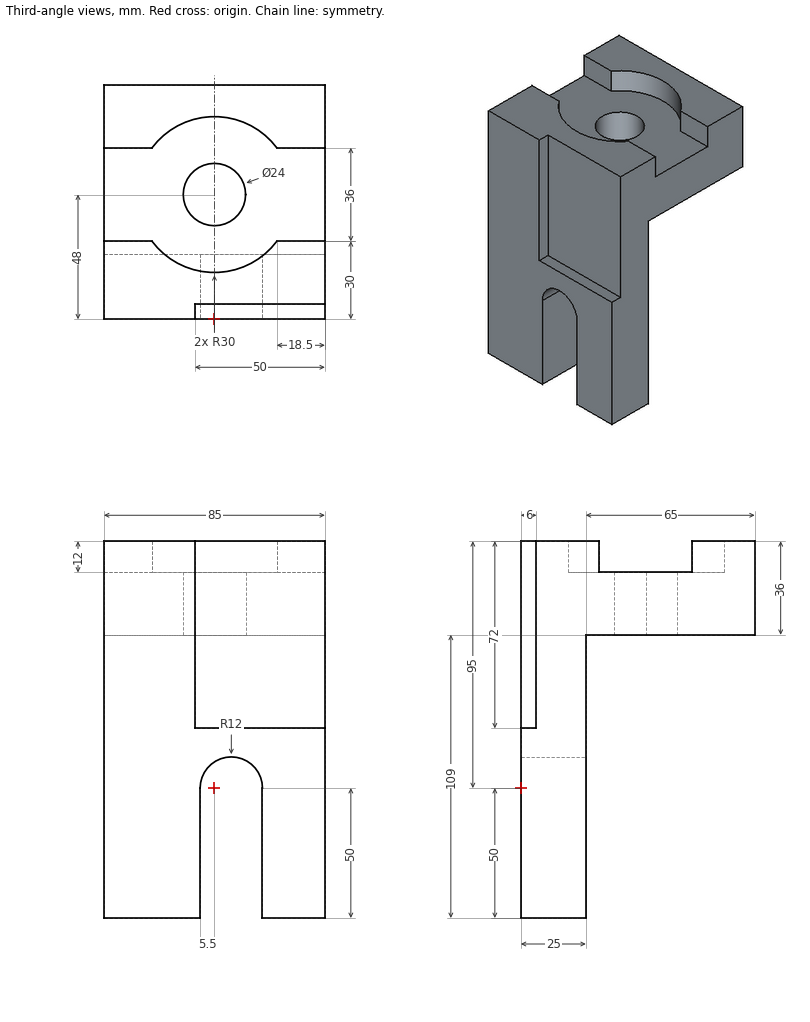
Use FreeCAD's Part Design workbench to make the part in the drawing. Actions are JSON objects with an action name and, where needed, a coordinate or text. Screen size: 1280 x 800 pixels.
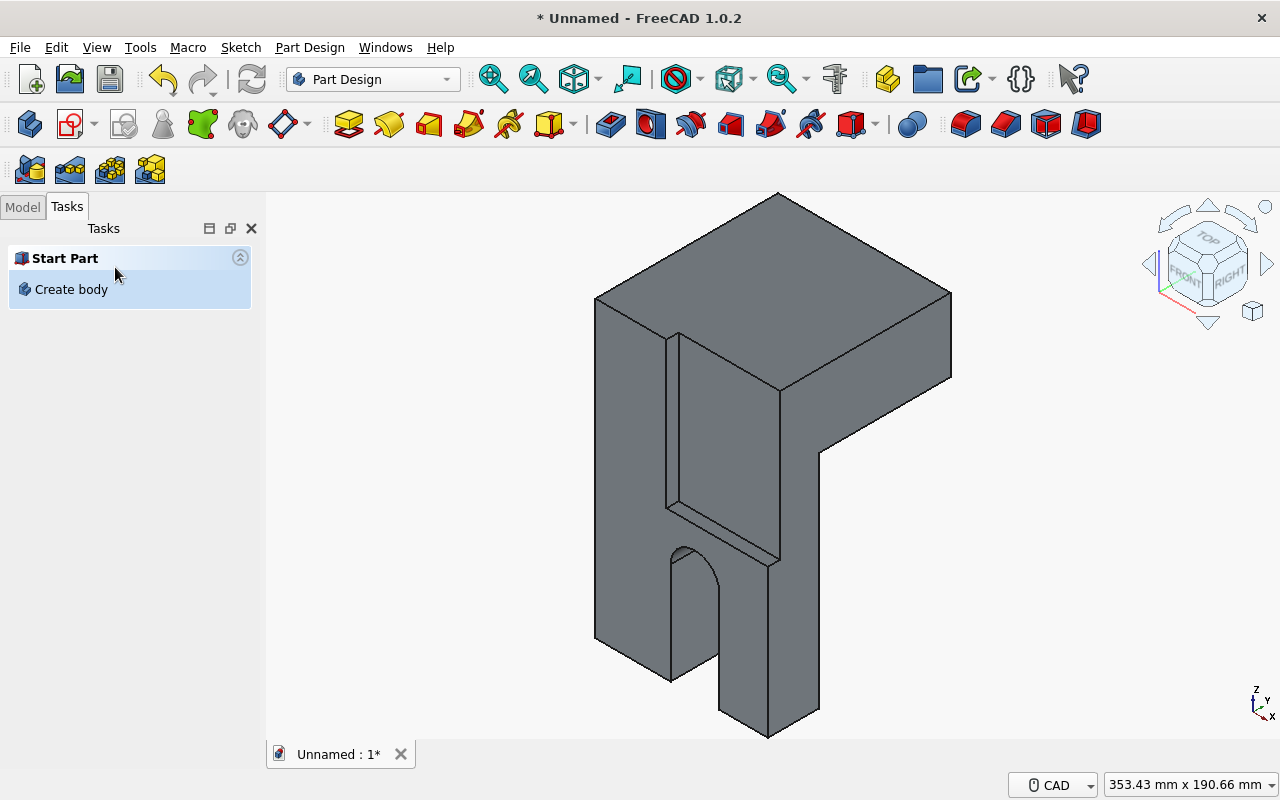
{"action": "left_click", "coordinate": [773, 295]}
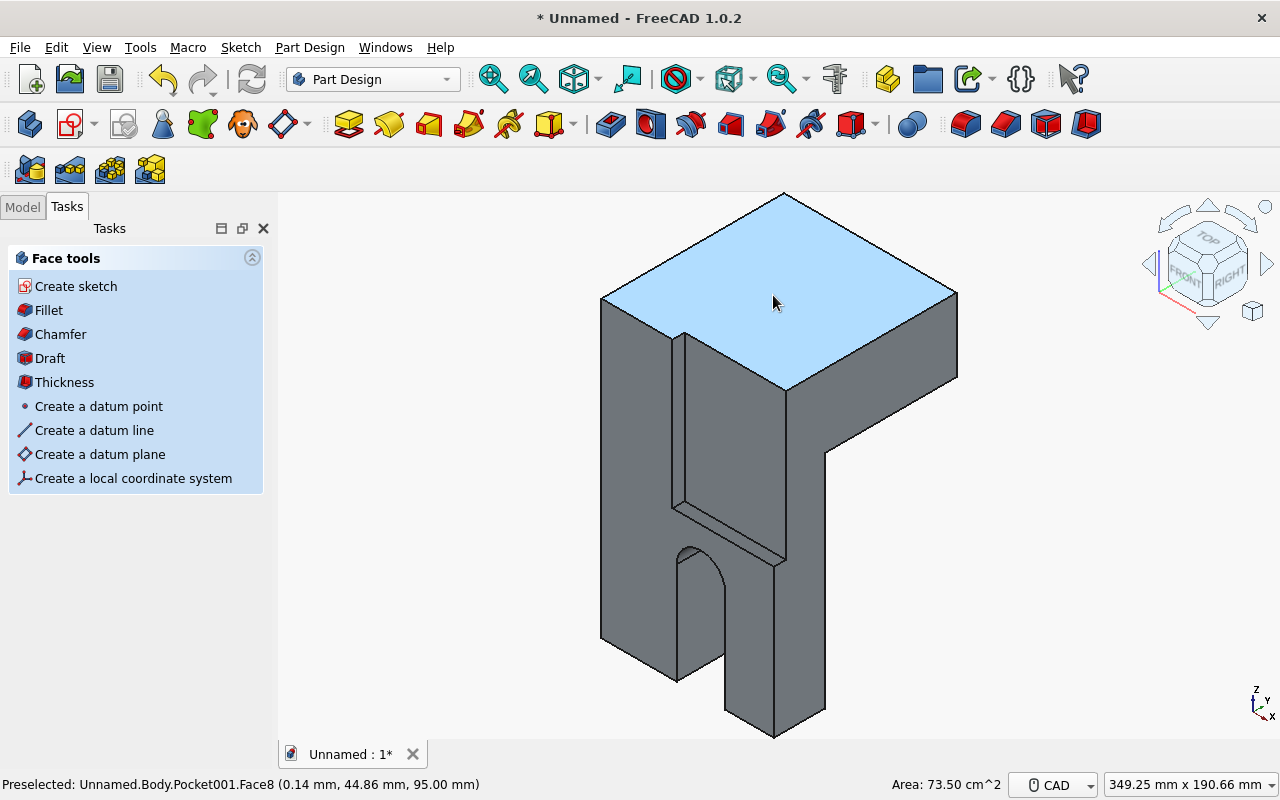
{"action": "left_click", "coordinate": [70, 124]}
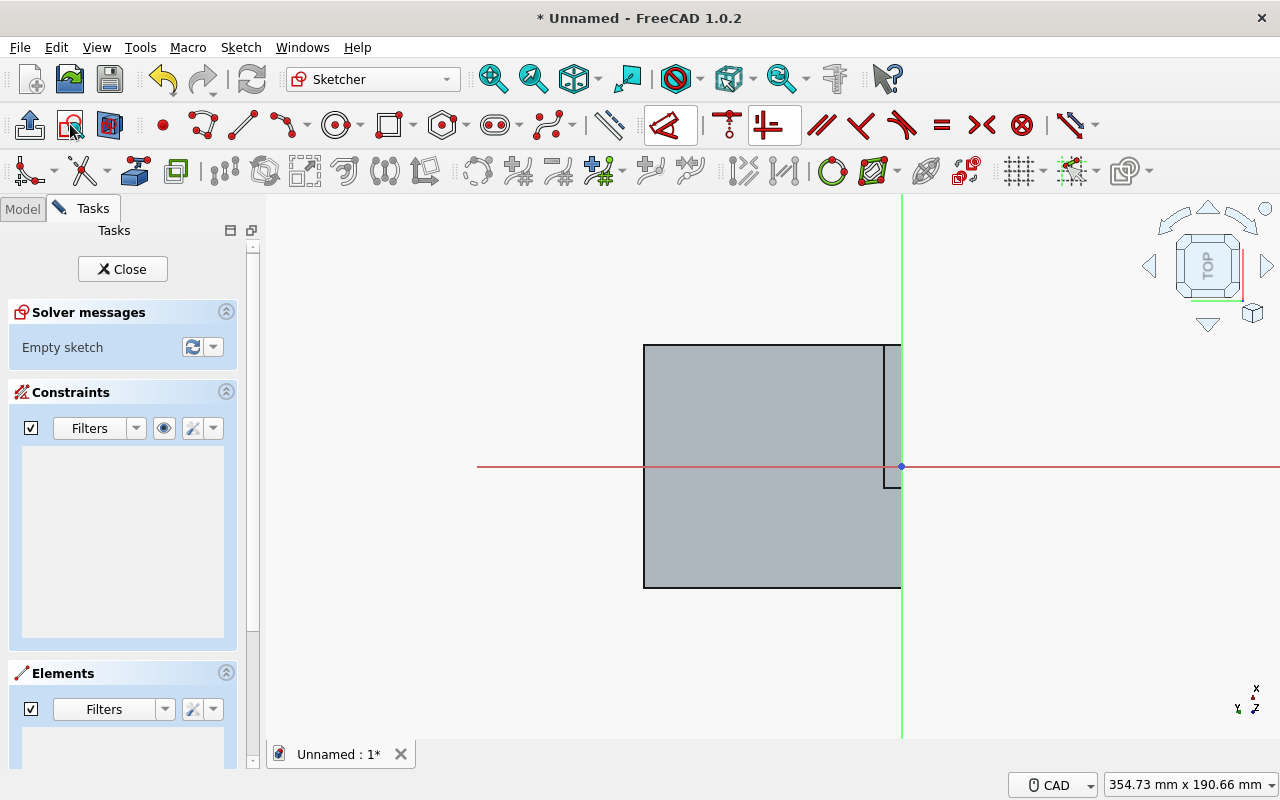
{"action": "scroll", "coordinate": [964, 467], "scroll_direction": "up", "scroll_amount": 2}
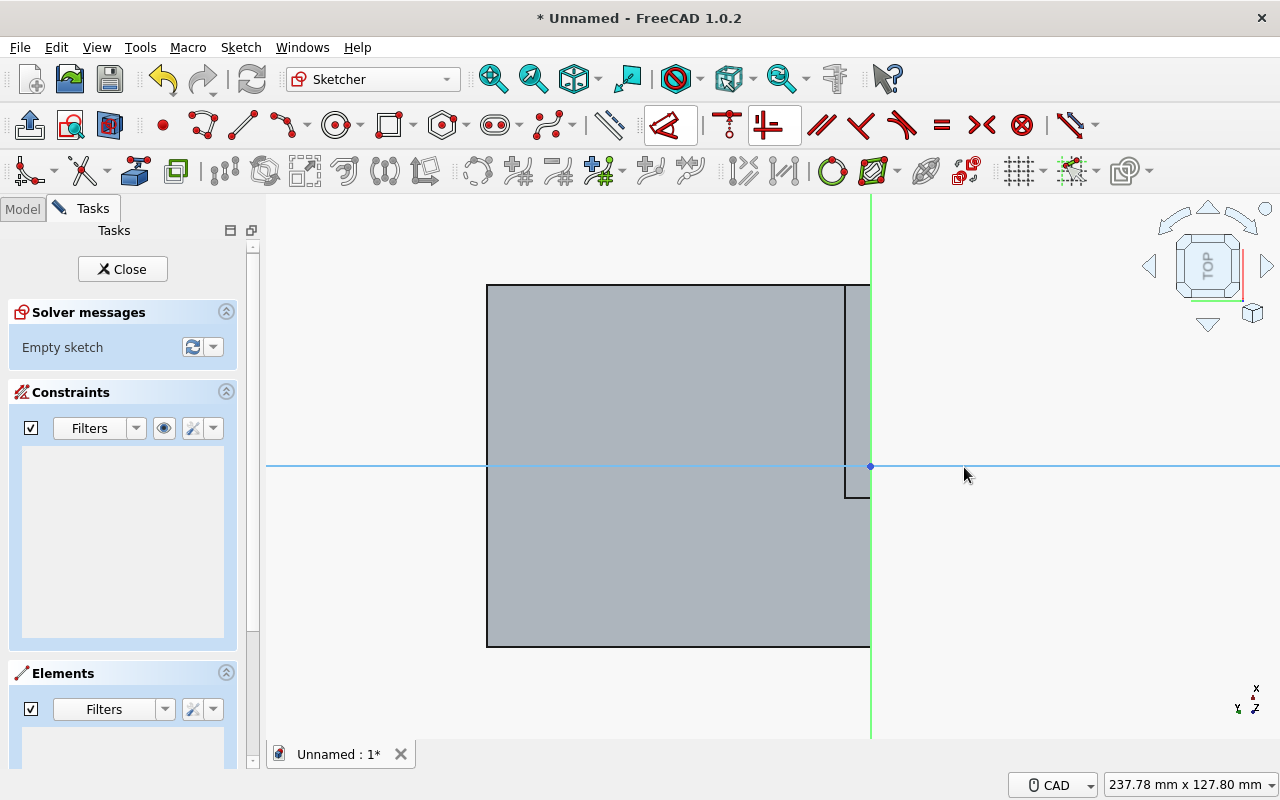
{"action": "left_click", "coordinate": [204, 126]}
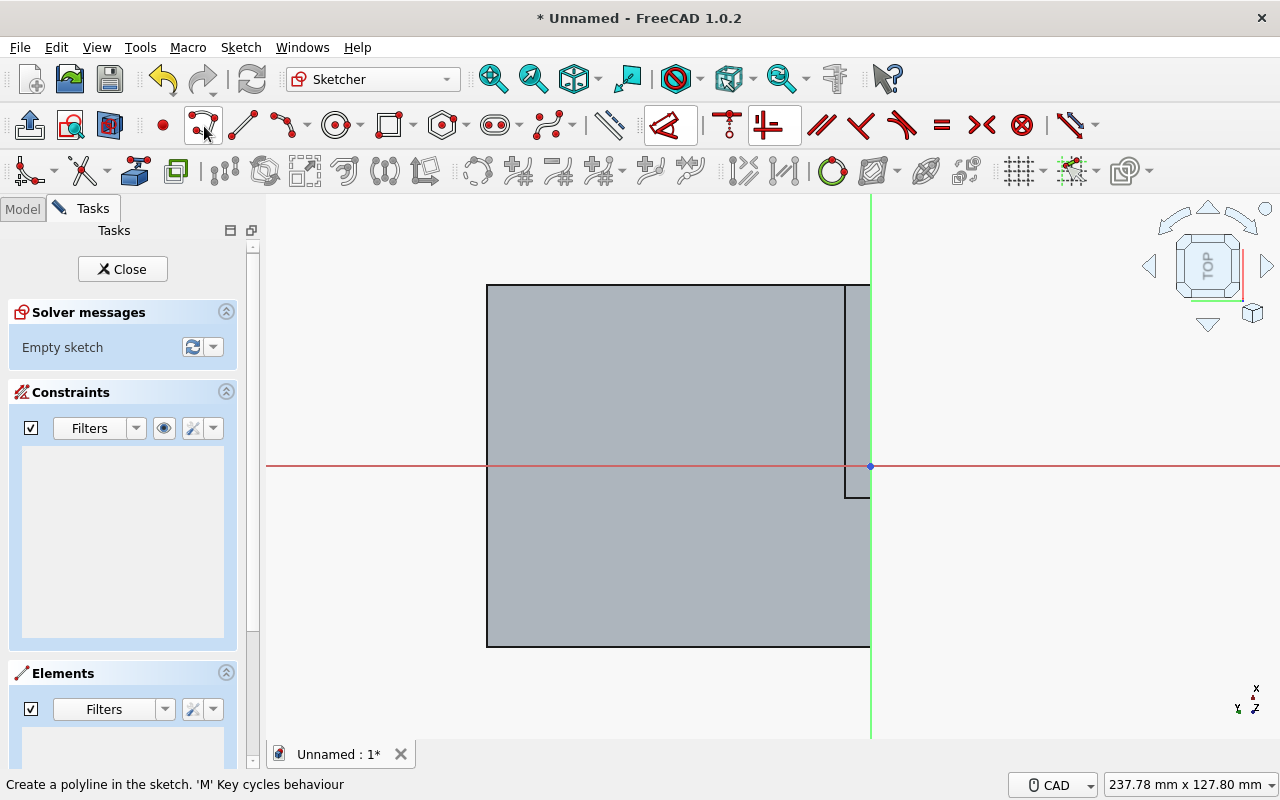
{"action": "left_click", "coordinate": [743, 364]}
{"action": "left_click", "coordinate": [743, 285]}
{"action": "left_click", "coordinate": [589, 285]}
{"action": "left_click", "coordinate": [589, 364]}
{"action": "right_click", "coordinate": [589, 364]}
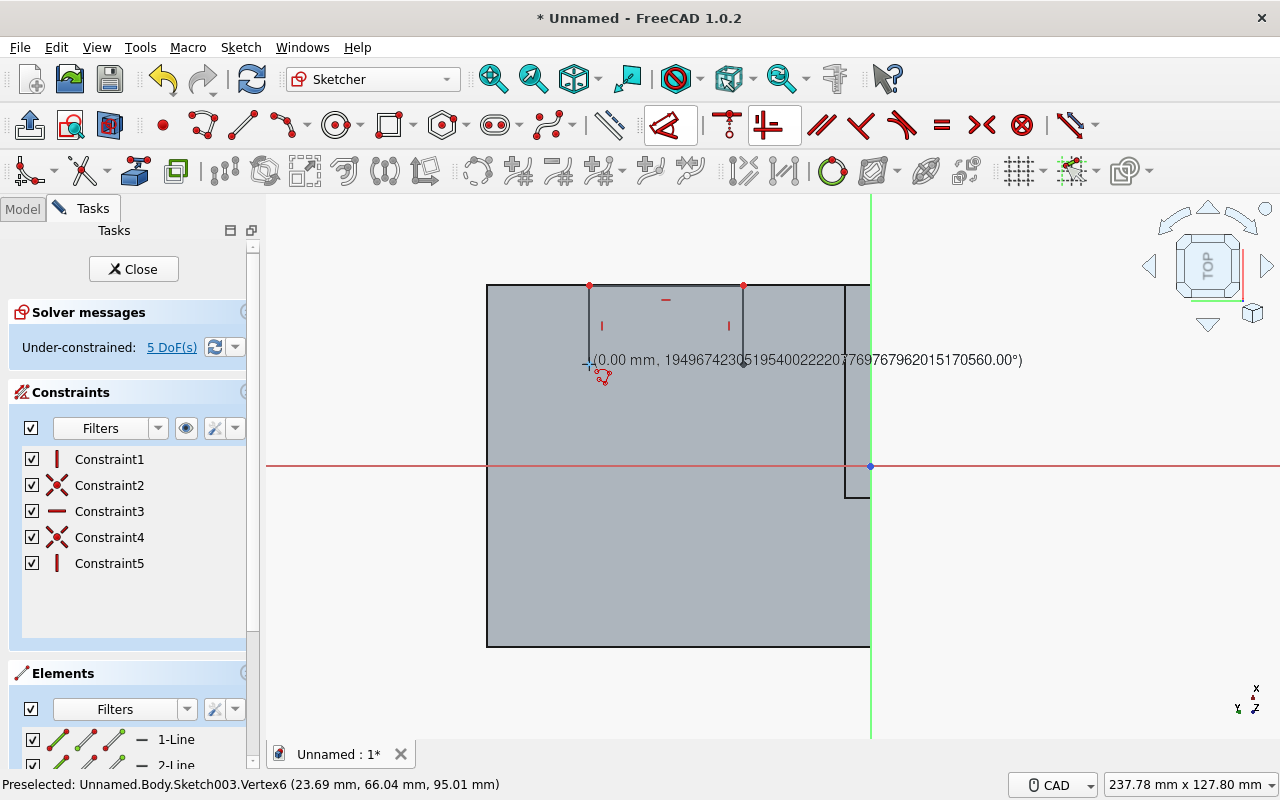
{"action": "left_click", "coordinate": [589, 568]}
{"action": "left_click", "coordinate": [589, 647]}
{"action": "left_click", "coordinate": [743, 647]}
{"action": "left_click", "coordinate": [743, 568]}
{"action": "right_click", "coordinate": [743, 568]}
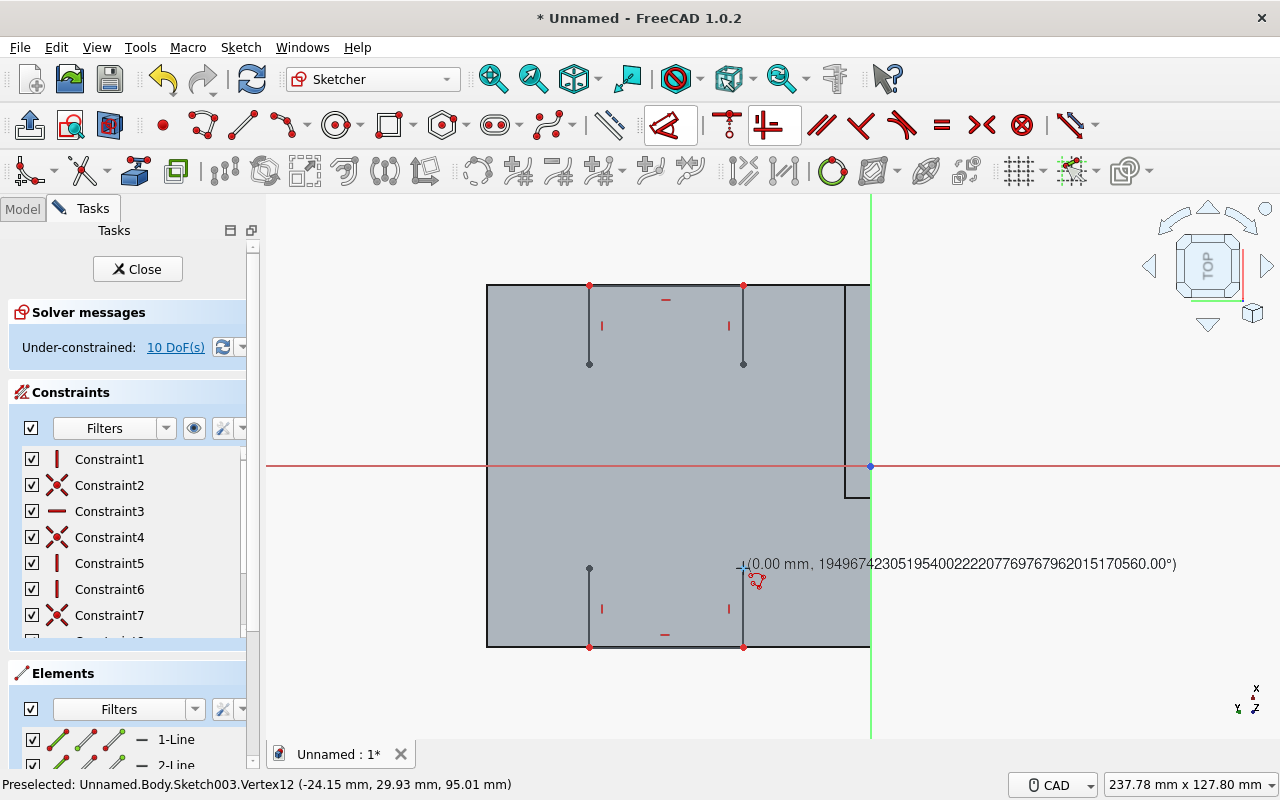
{"action": "left_click", "coordinate": [284, 126]}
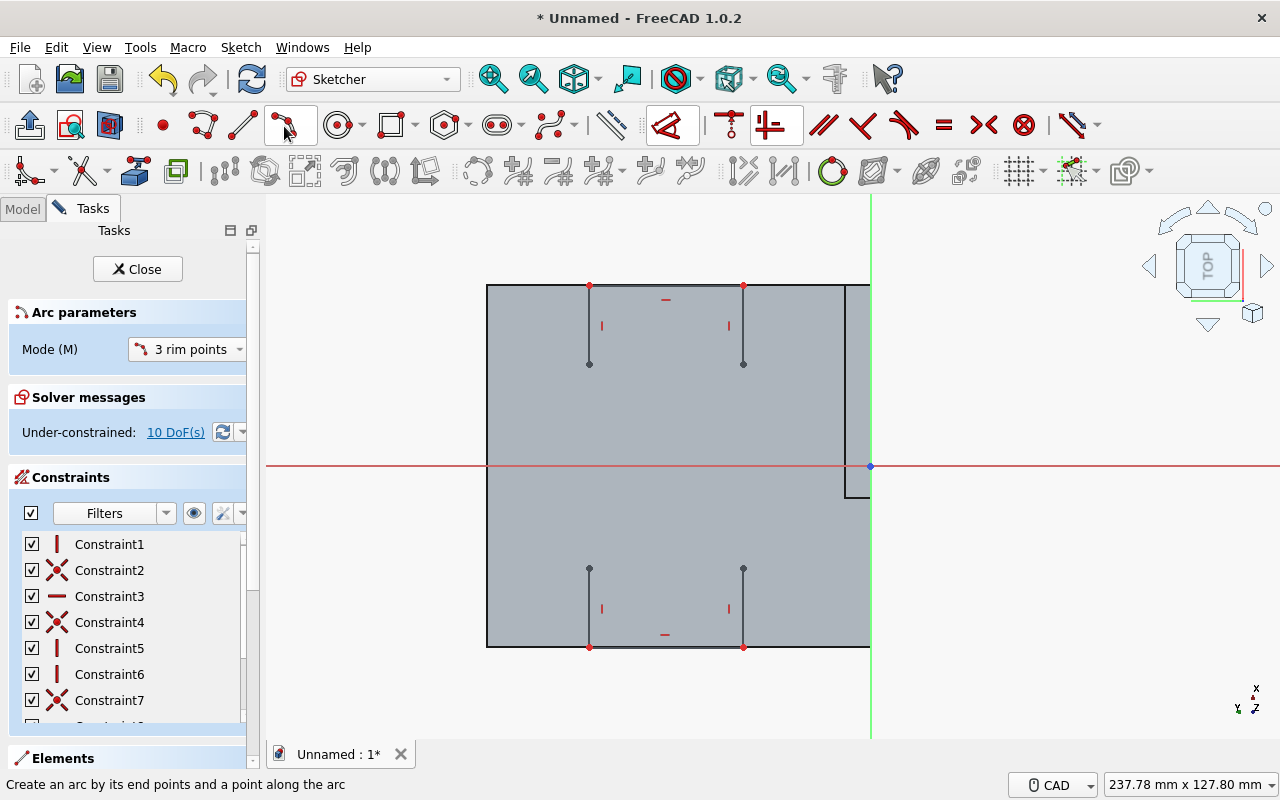
{"action": "left_click", "coordinate": [589, 365]}
{"action": "left_click", "coordinate": [589, 569]}
{"action": "left_click", "coordinate": [540, 442]}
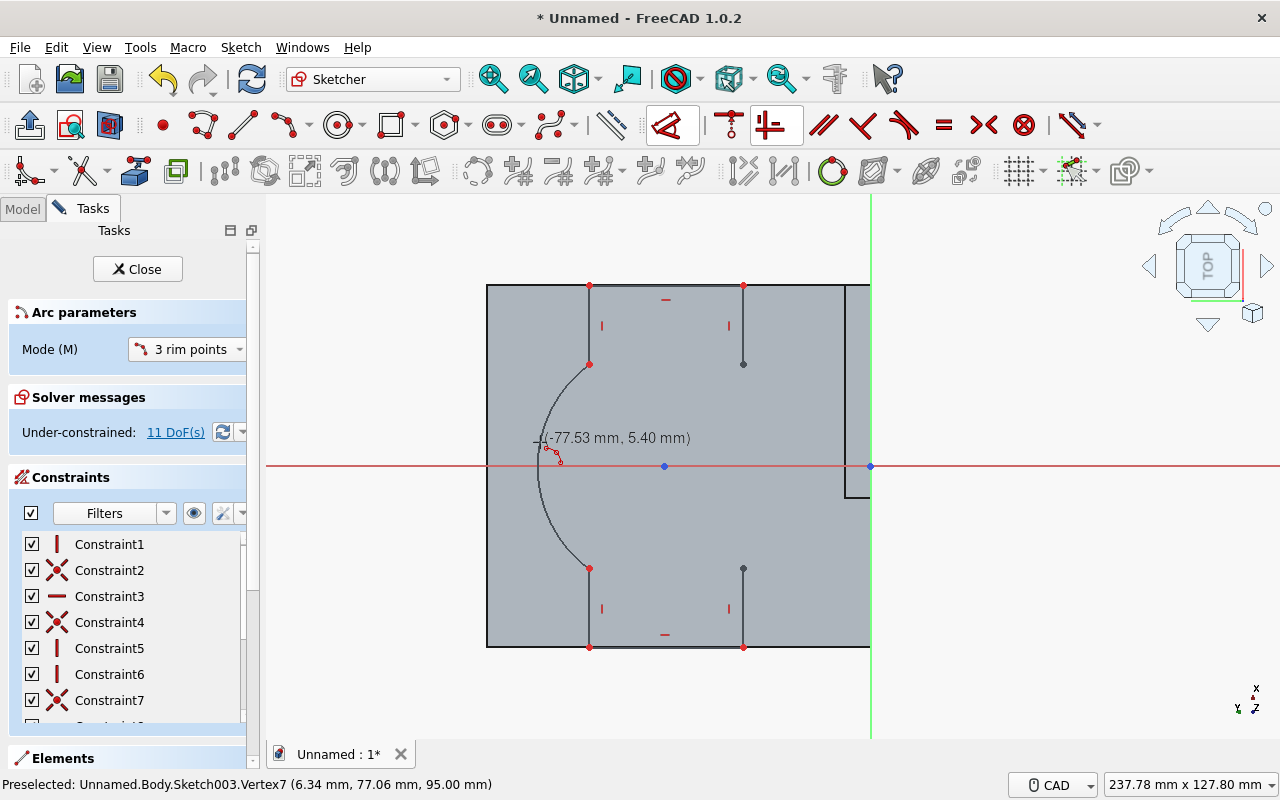
{"action": "left_click", "coordinate": [743, 569]}
{"action": "left_click", "coordinate": [743, 365]}
{"action": "left_click", "coordinate": [792, 490]}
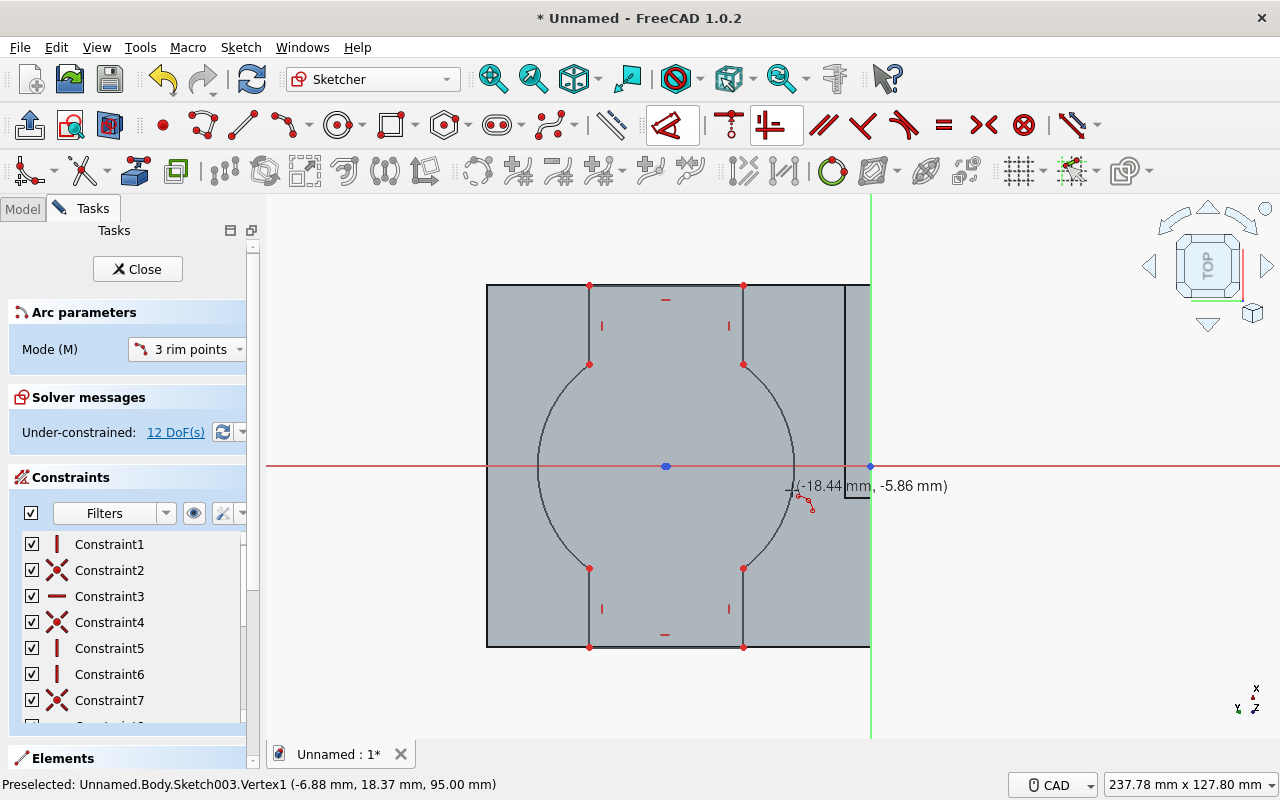
{"action": "left_click", "coordinate": [338, 126]}